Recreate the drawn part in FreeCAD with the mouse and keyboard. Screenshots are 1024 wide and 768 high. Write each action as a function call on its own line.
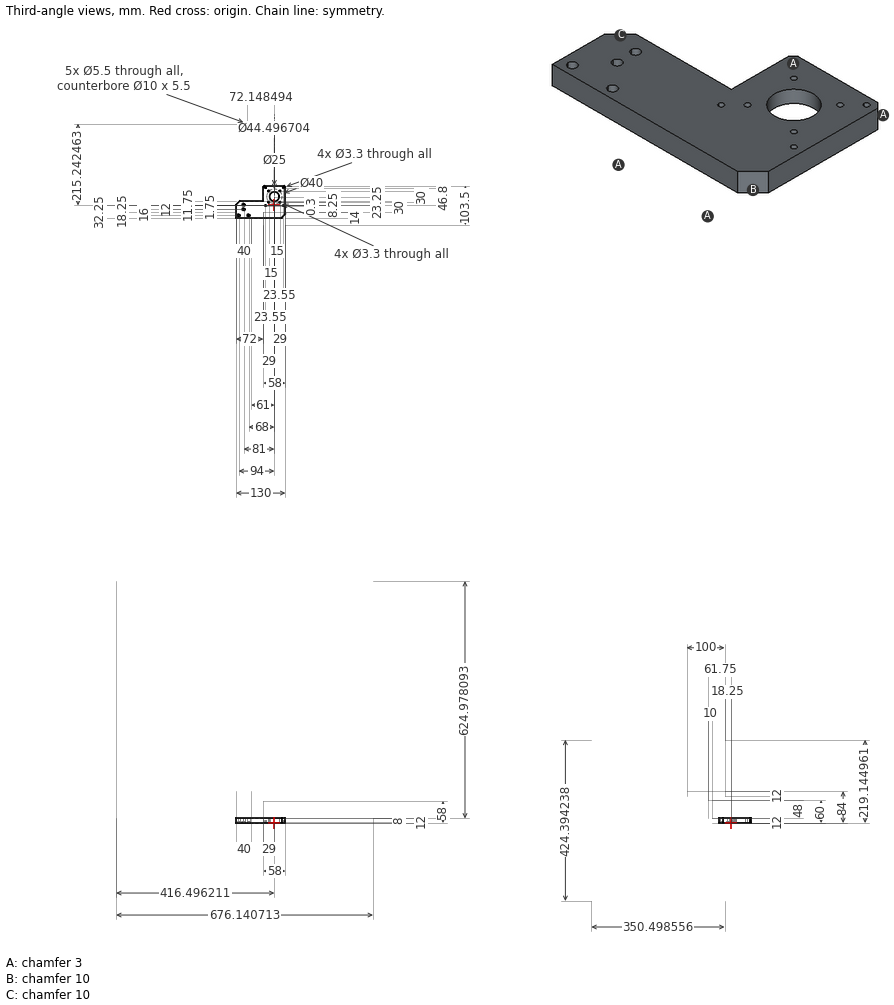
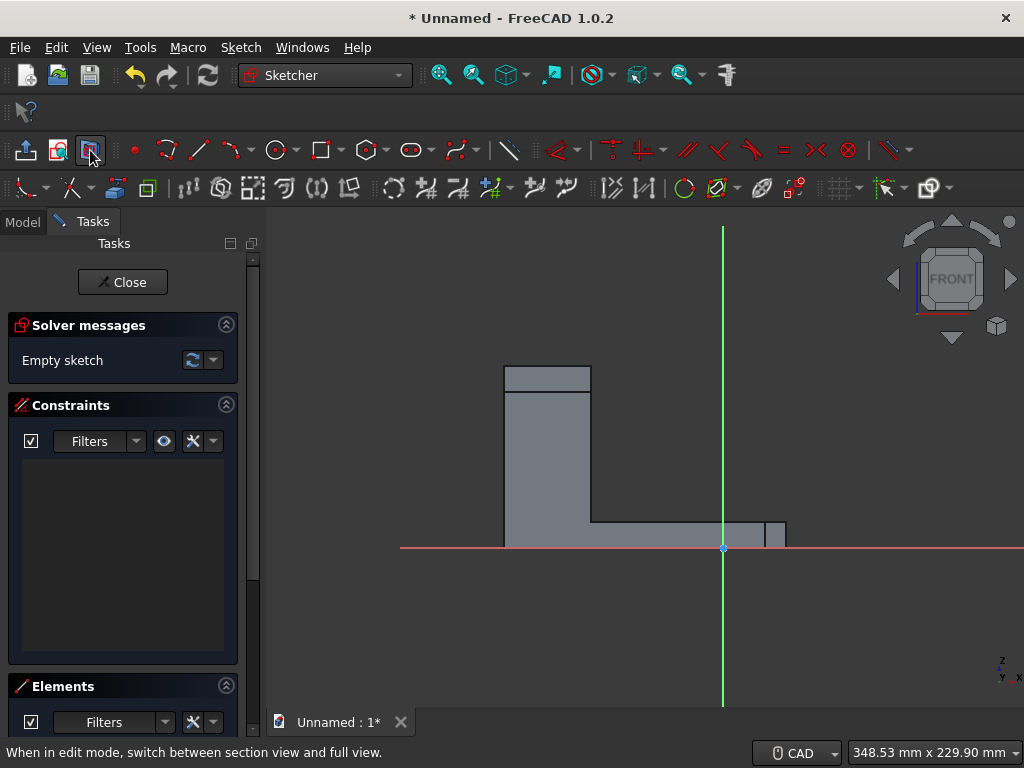
scroll(584, 654, down, 7)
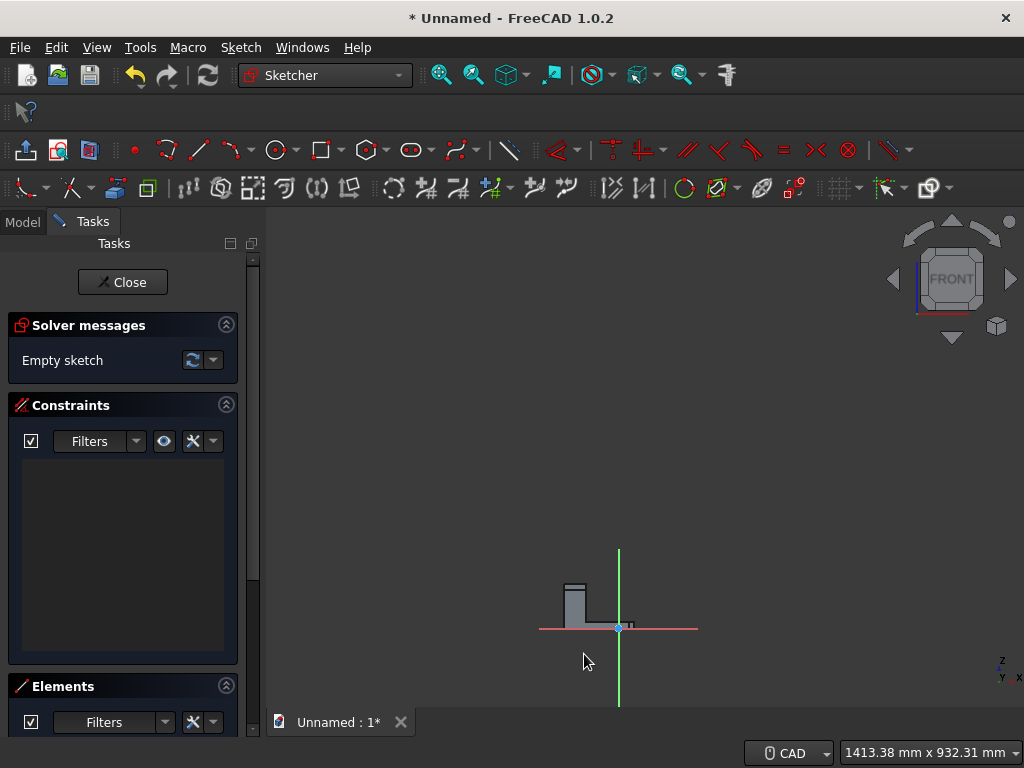
key(g)
key(r)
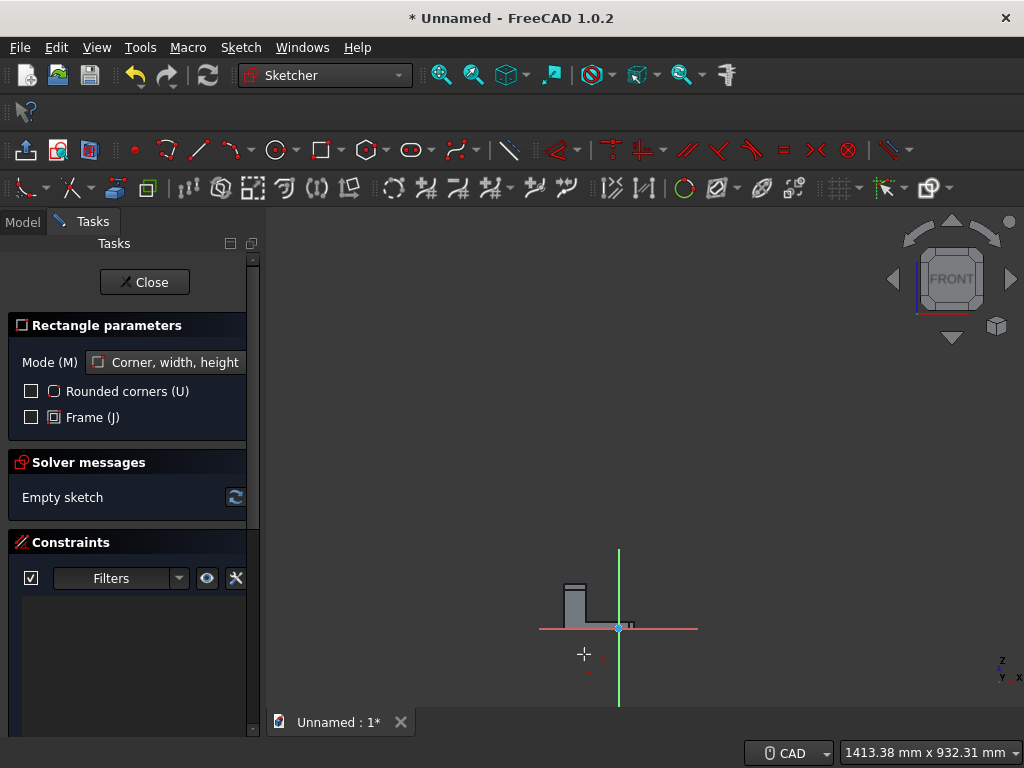
click(395, 287)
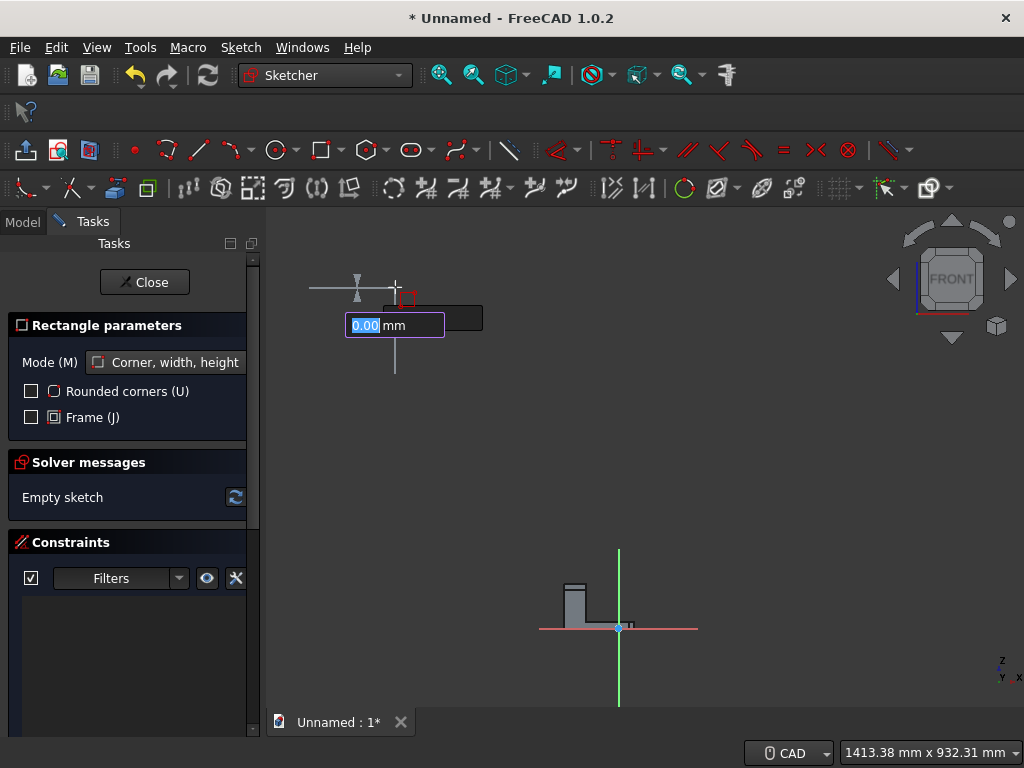
scroll(758, 622, up, 5)
move(757, 621)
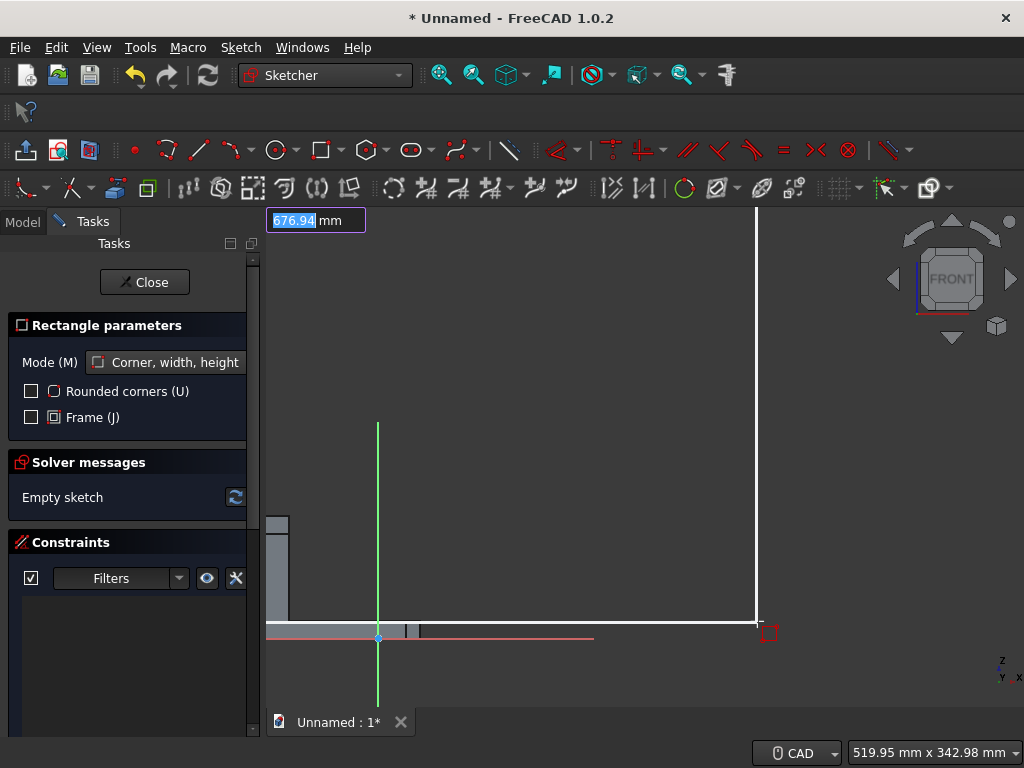
text(676.140713)
key(Tab)
text(624.978093)
key(Return)
key(Escape)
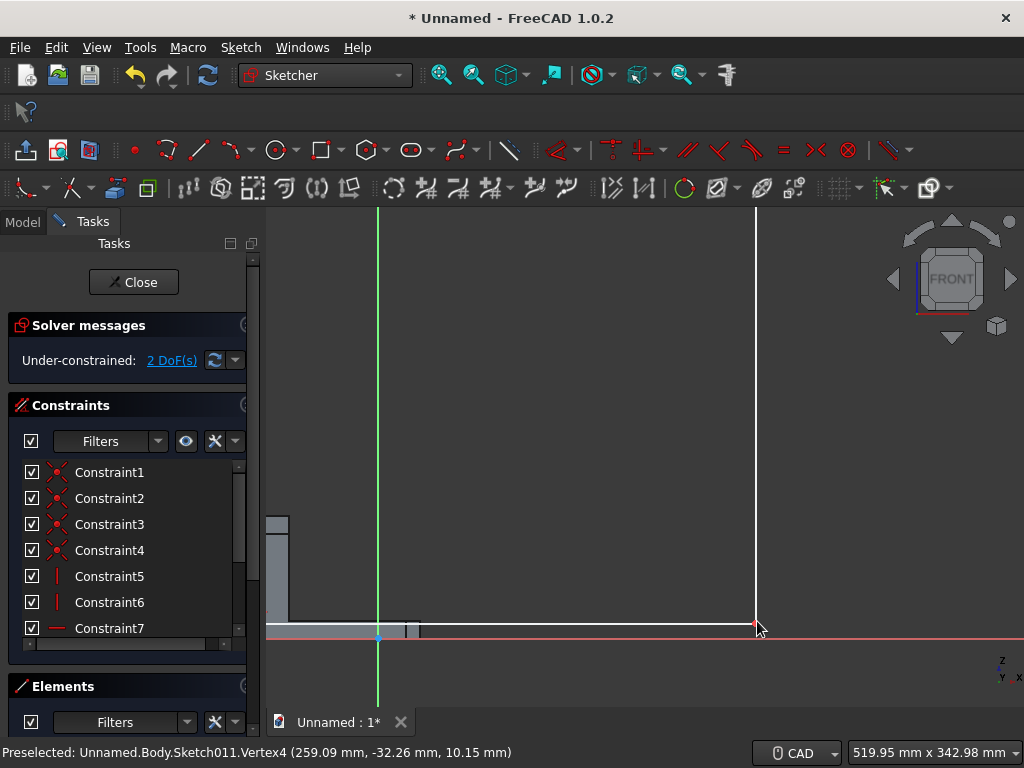
click(556, 150)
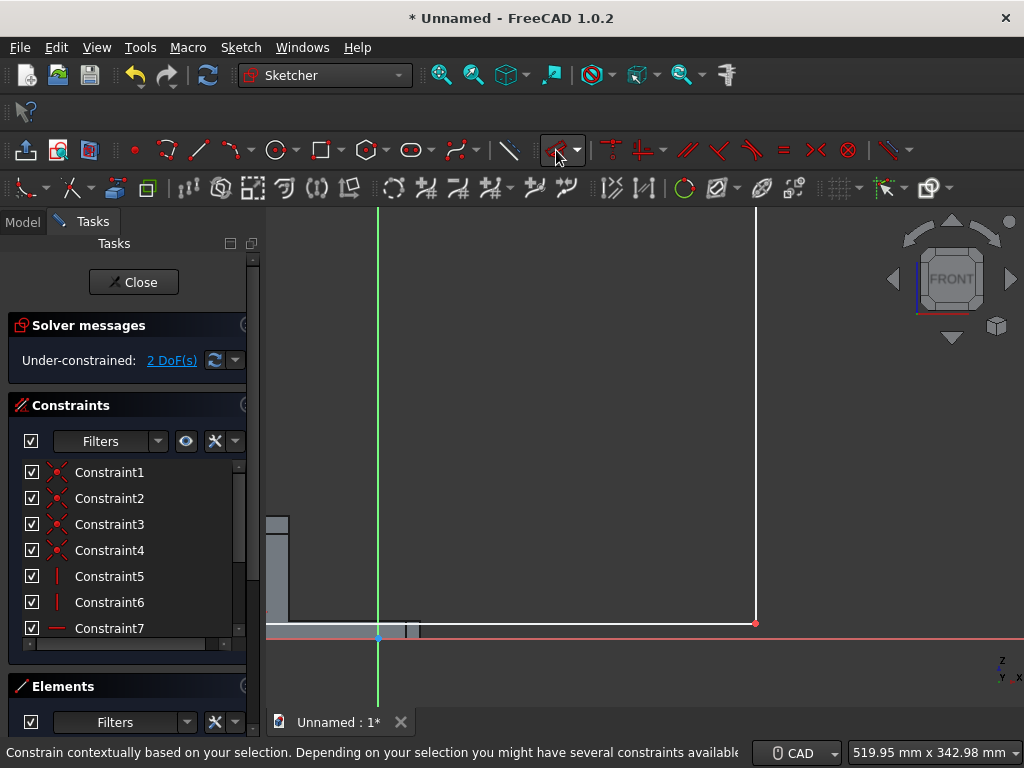
scroll(758, 622, down, 5)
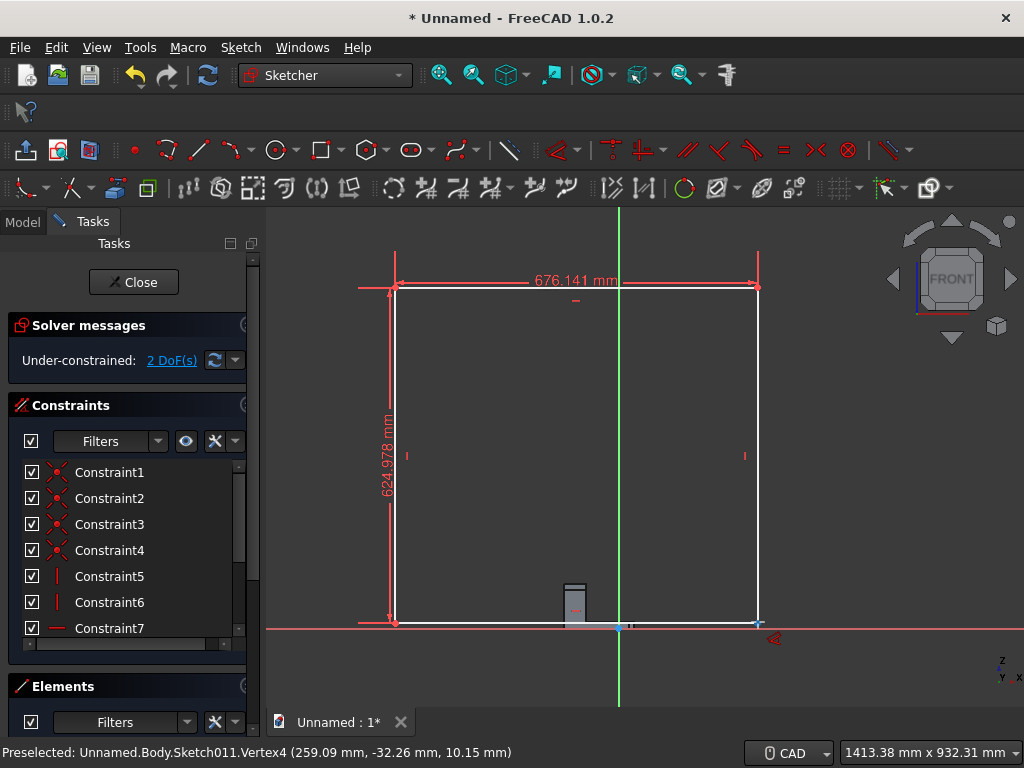
scroll(395, 623, up, 10)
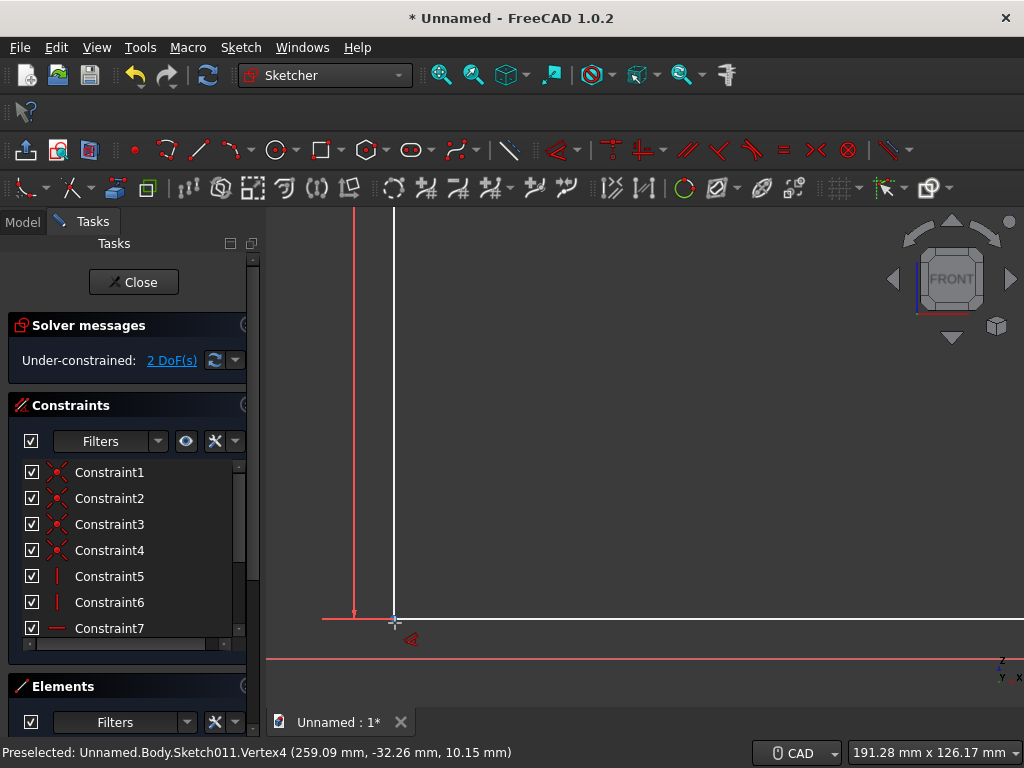
click(394, 619)
click(360, 639)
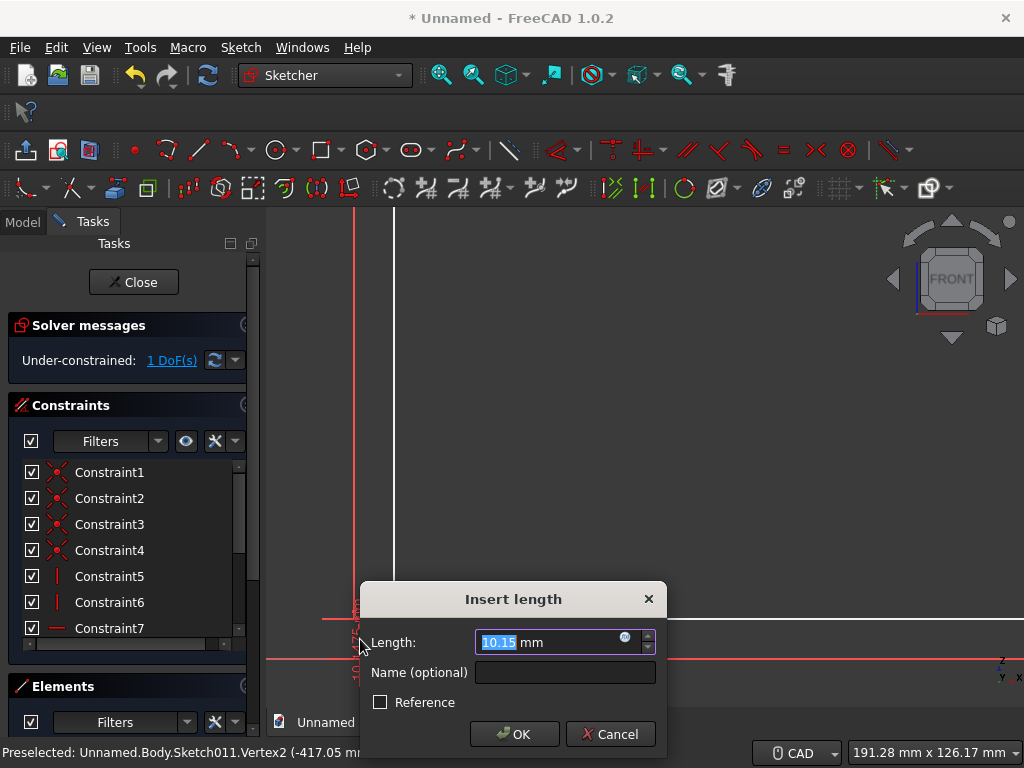
text(12)
key(Return)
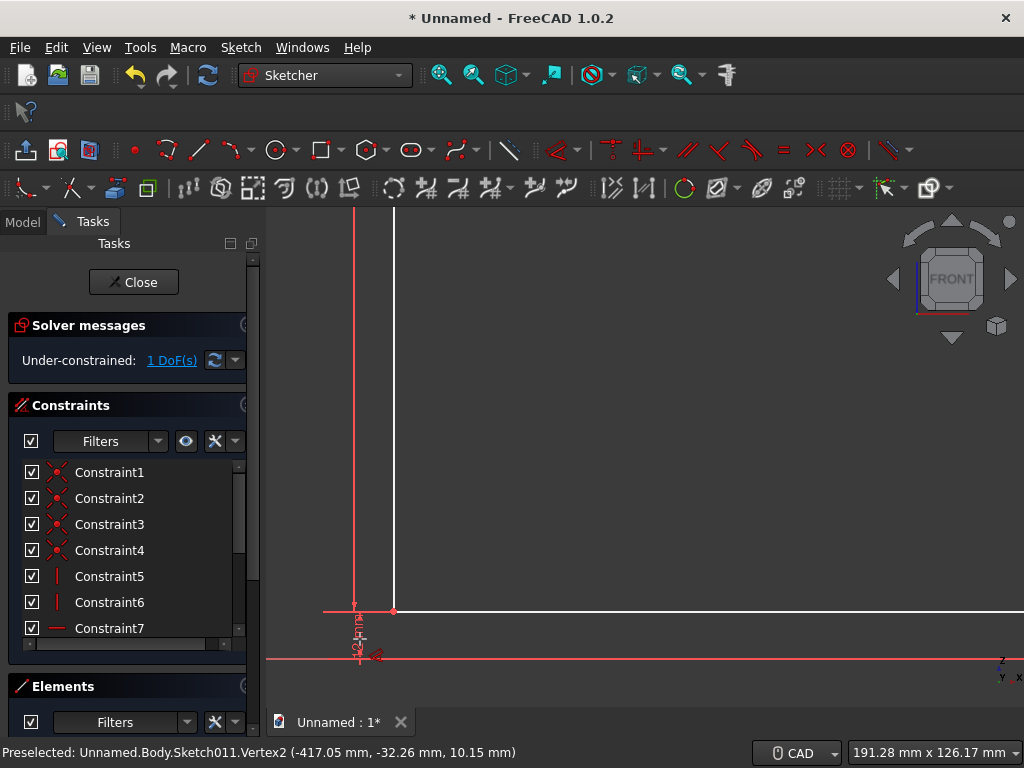
scroll(395, 623, down, 10)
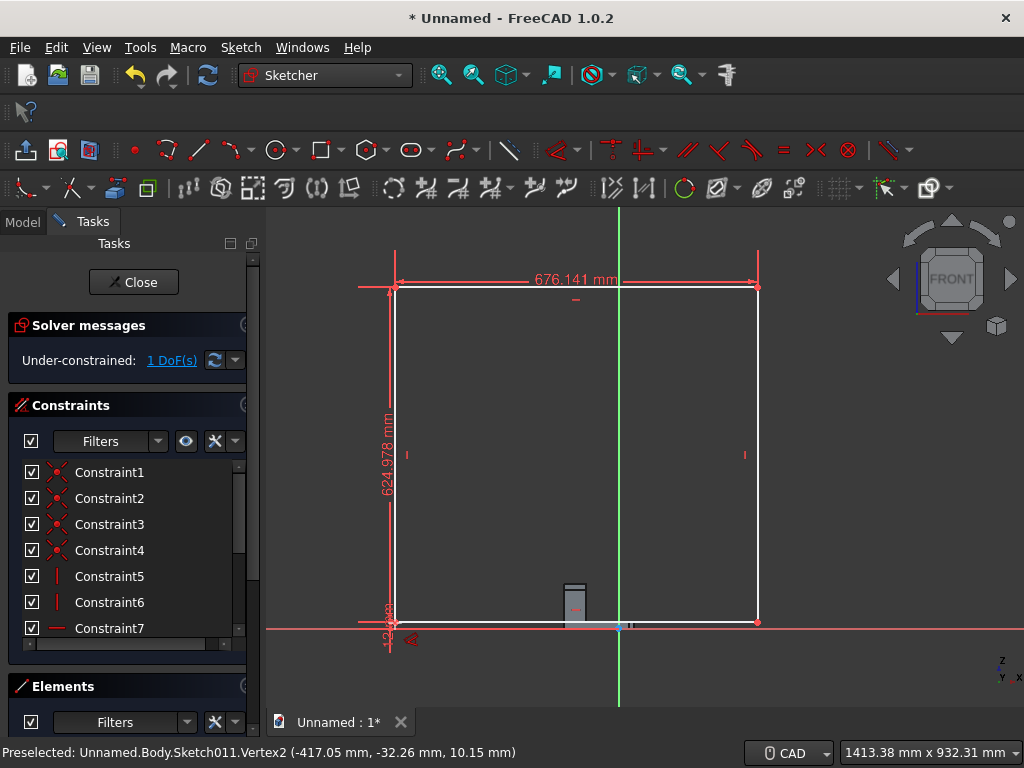
click(395, 287)
click(507, 253)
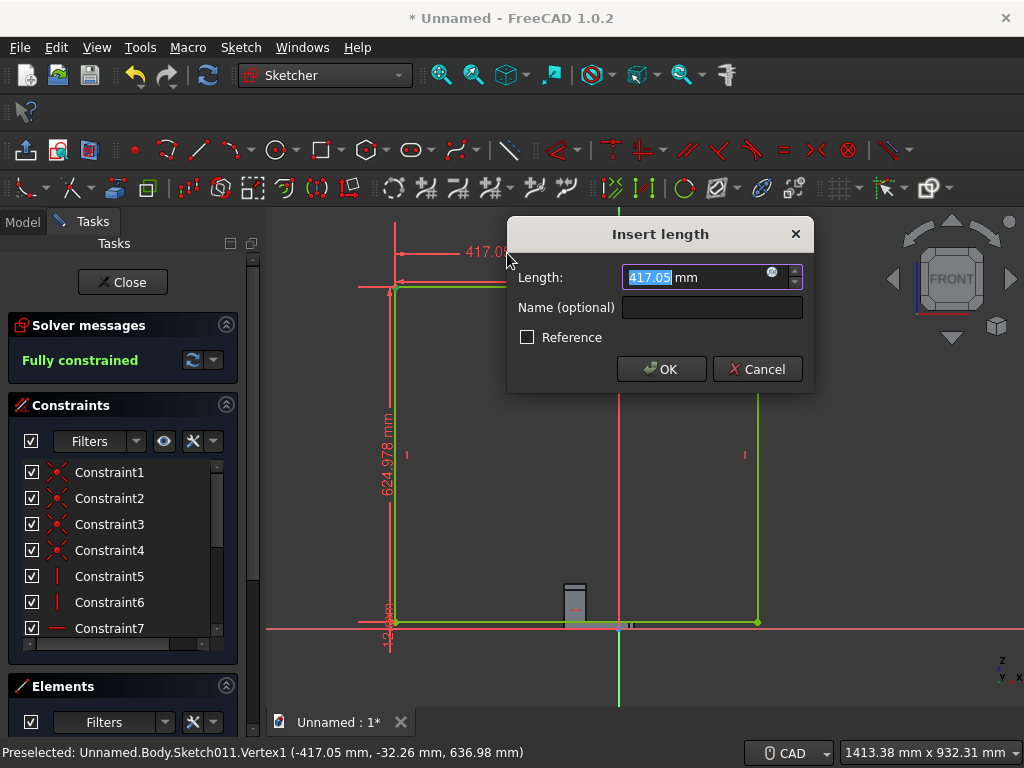
text(416.496211)
key(Return)
key(Escape)